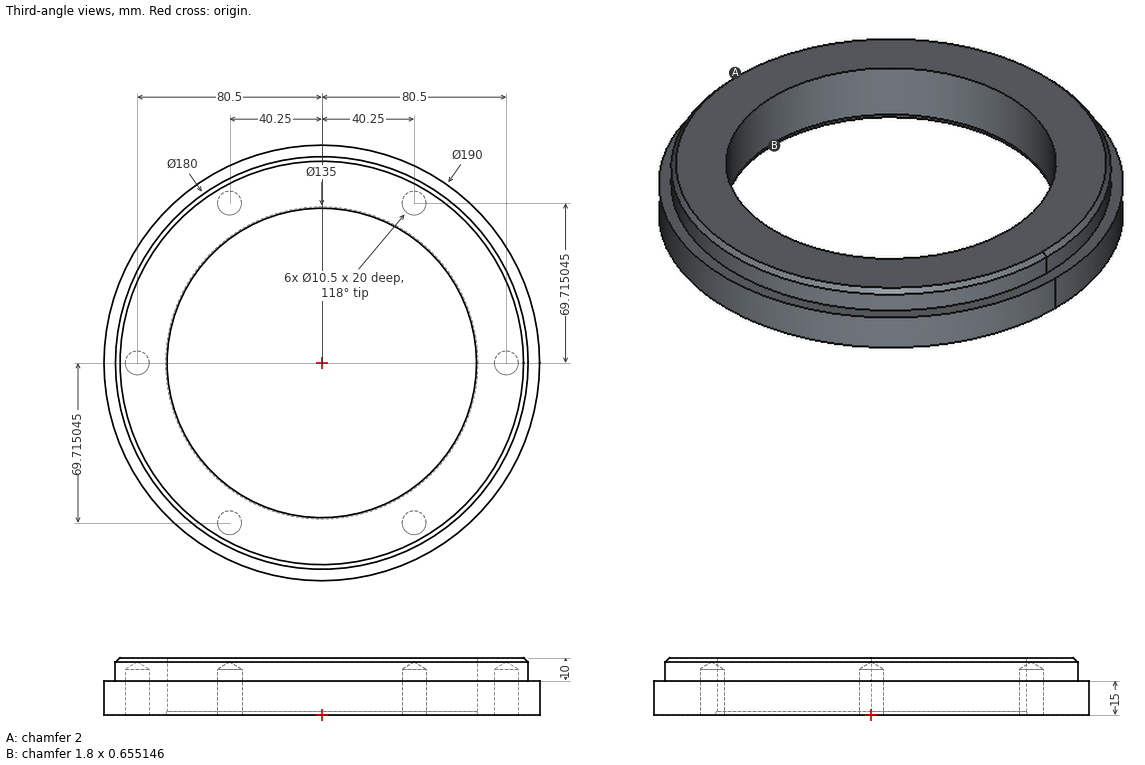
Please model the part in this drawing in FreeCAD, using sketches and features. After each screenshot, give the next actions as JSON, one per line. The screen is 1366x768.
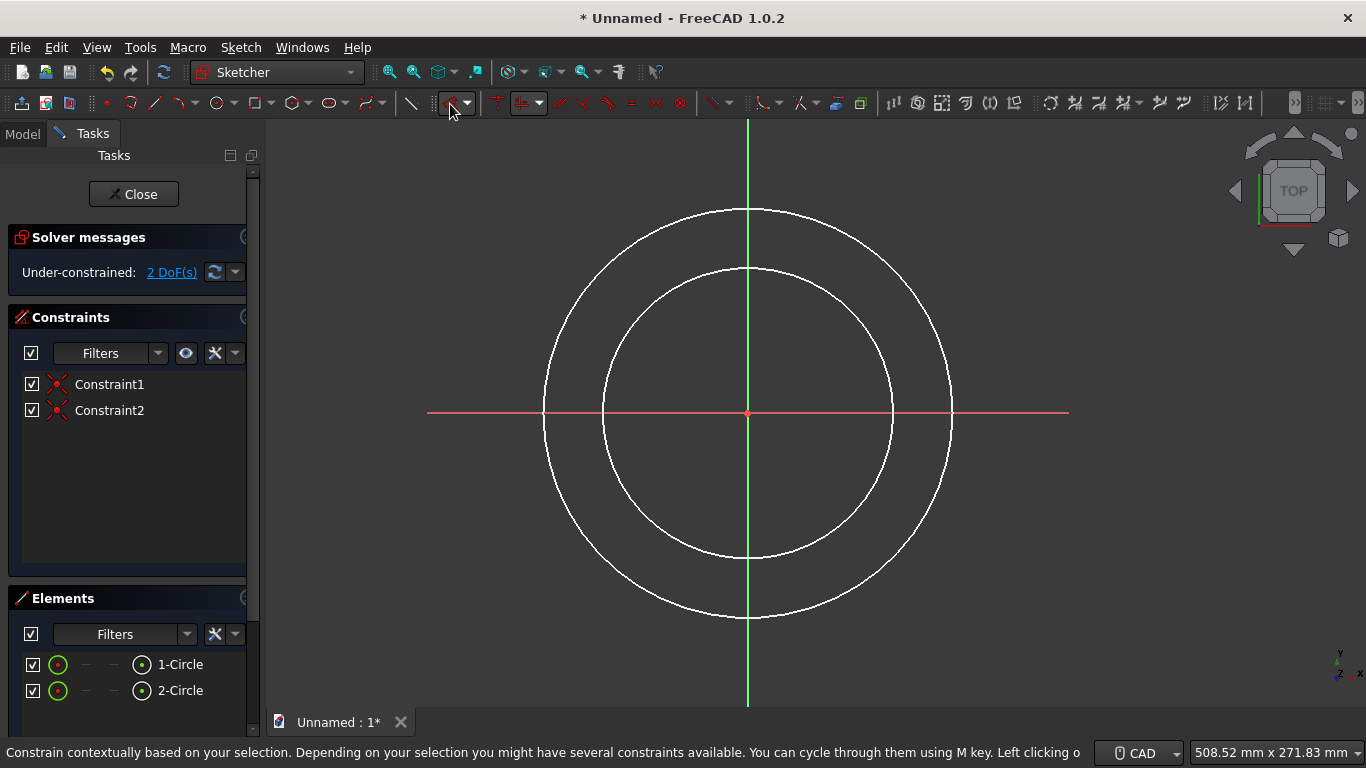
{"action": "left_click", "coordinate": [892, 268]}
{"action": "left_click", "coordinate": [915, 245]}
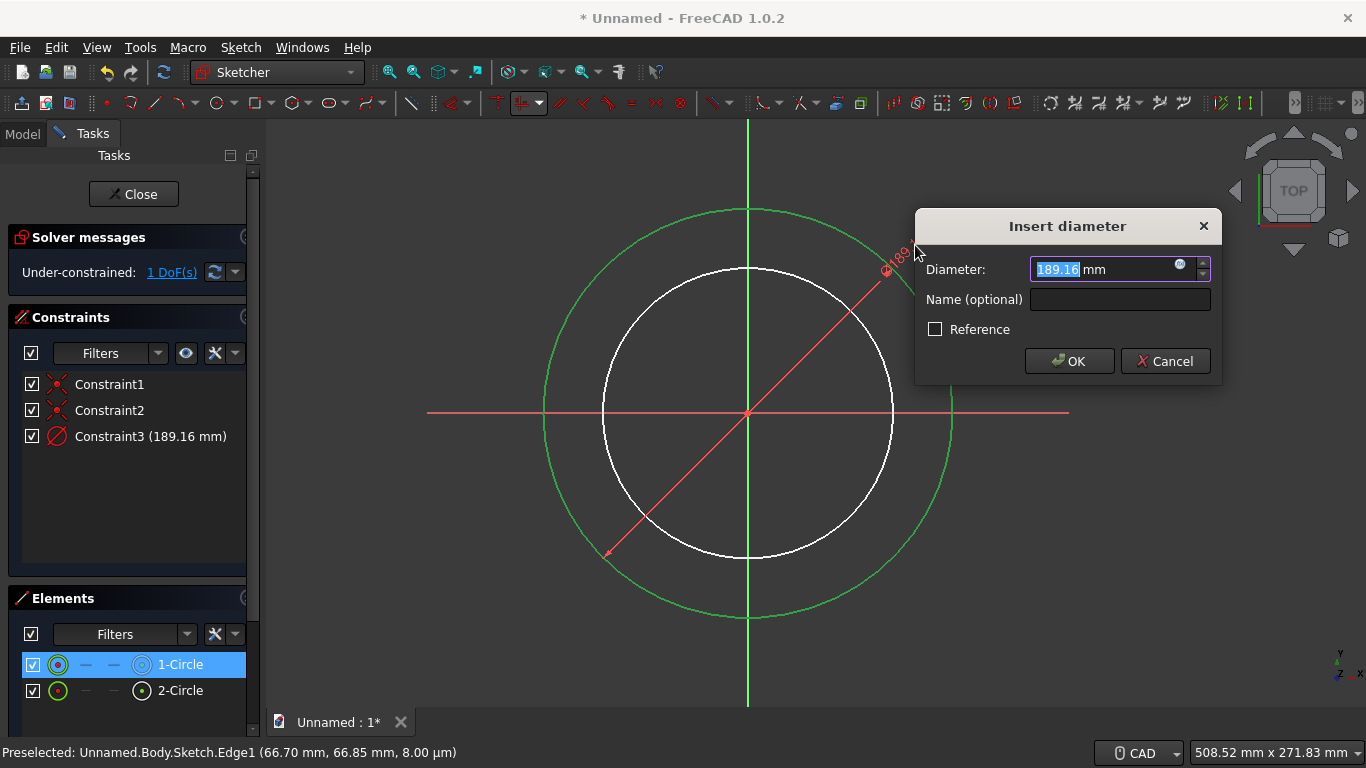
{"action": "type", "text": "190"}
{"action": "key", "text": "Return"}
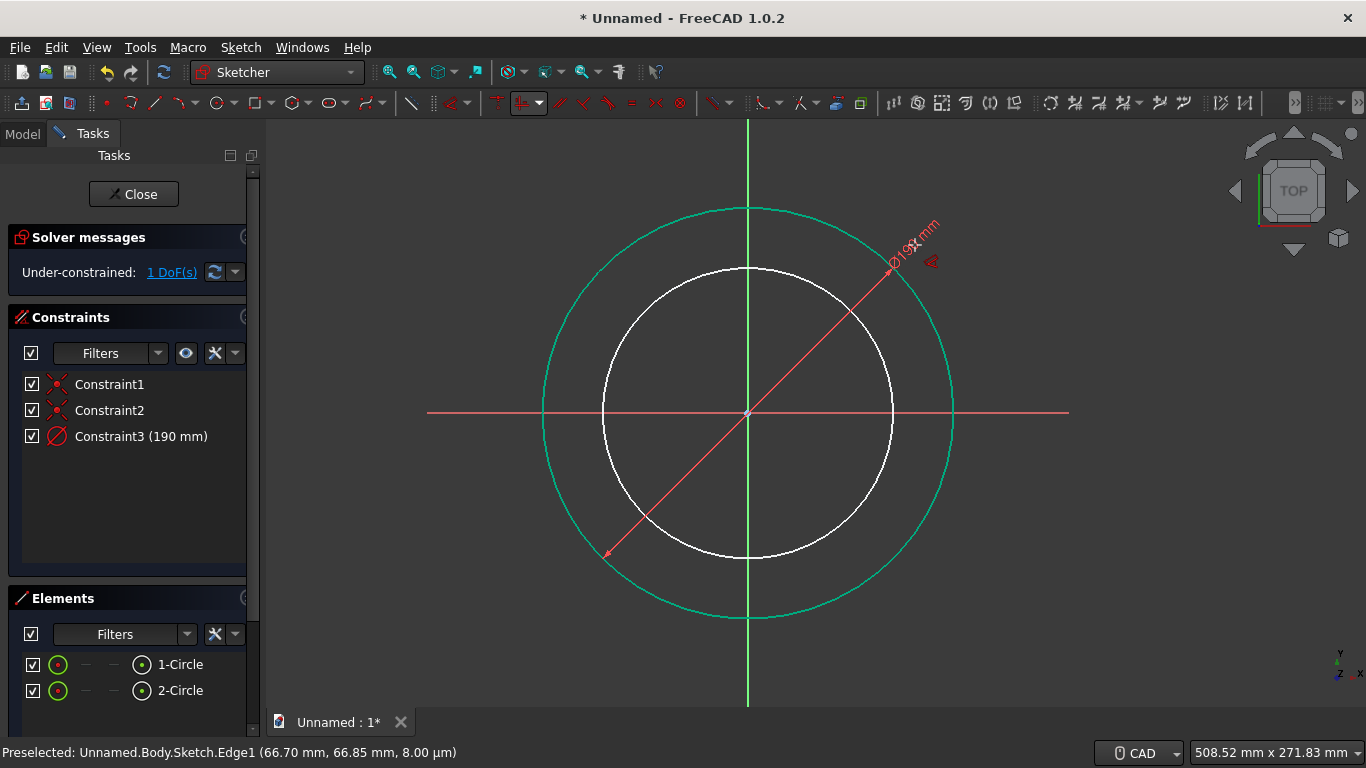
{"action": "left_click", "coordinate": [850, 310]}
{"action": "left_click", "coordinate": [872, 287]}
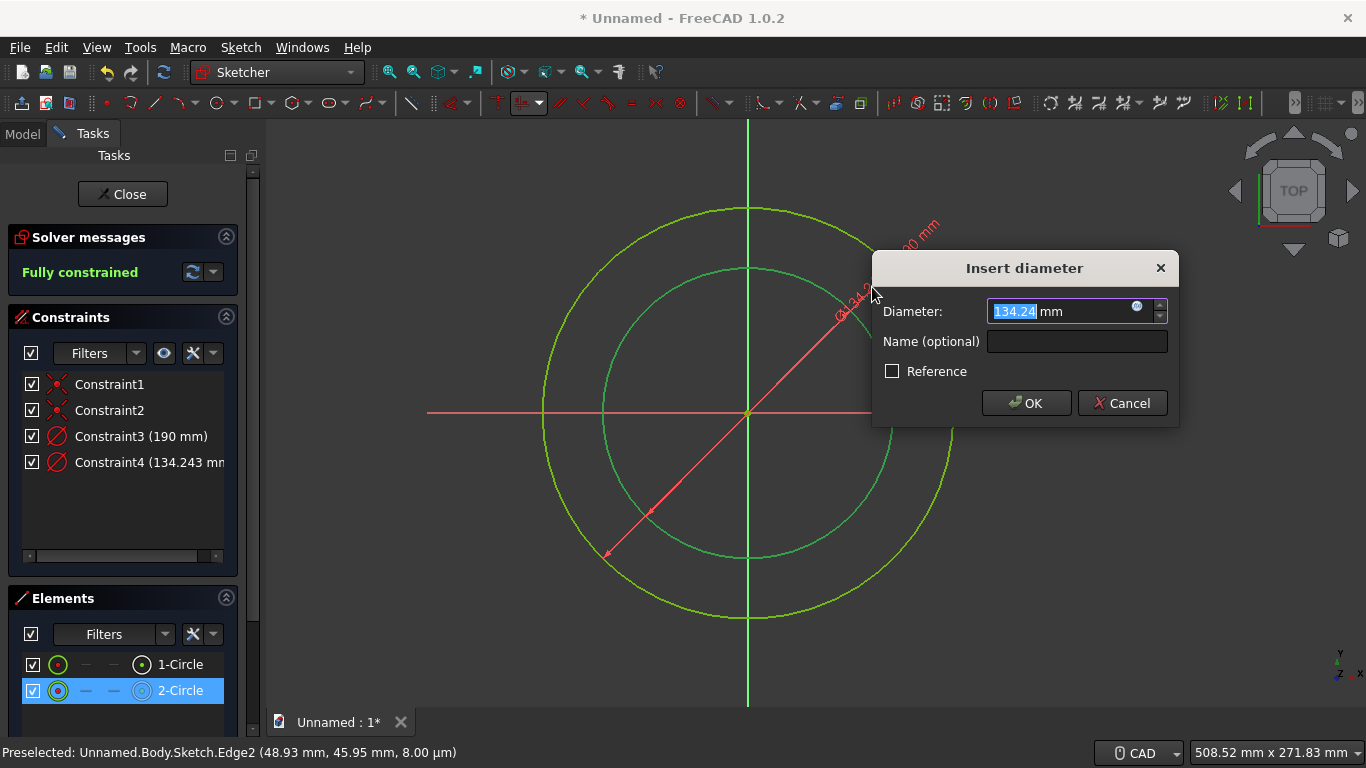
{"action": "type", "text": "135"}
{"action": "key", "text": "Return"}
{"action": "key", "text": "Escape"}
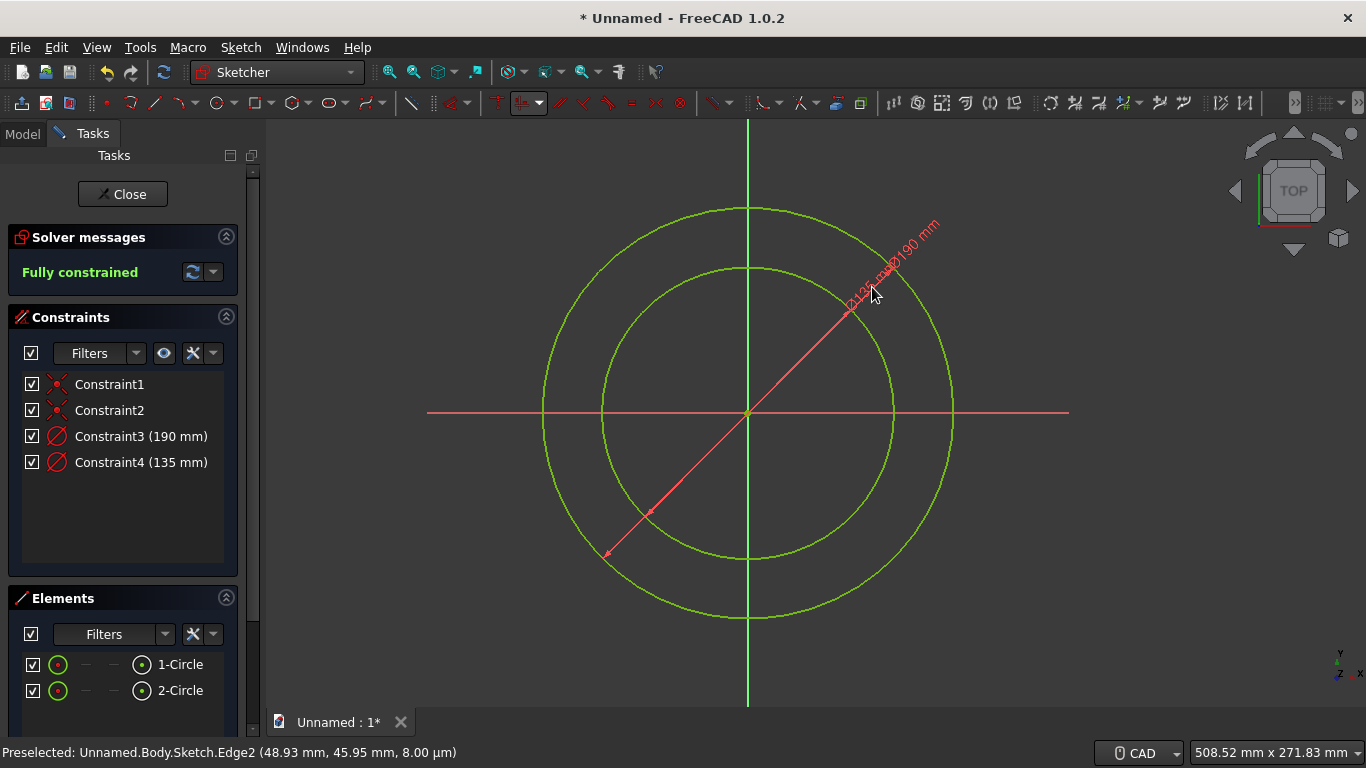
{"action": "left_click", "coordinate": [123, 194]}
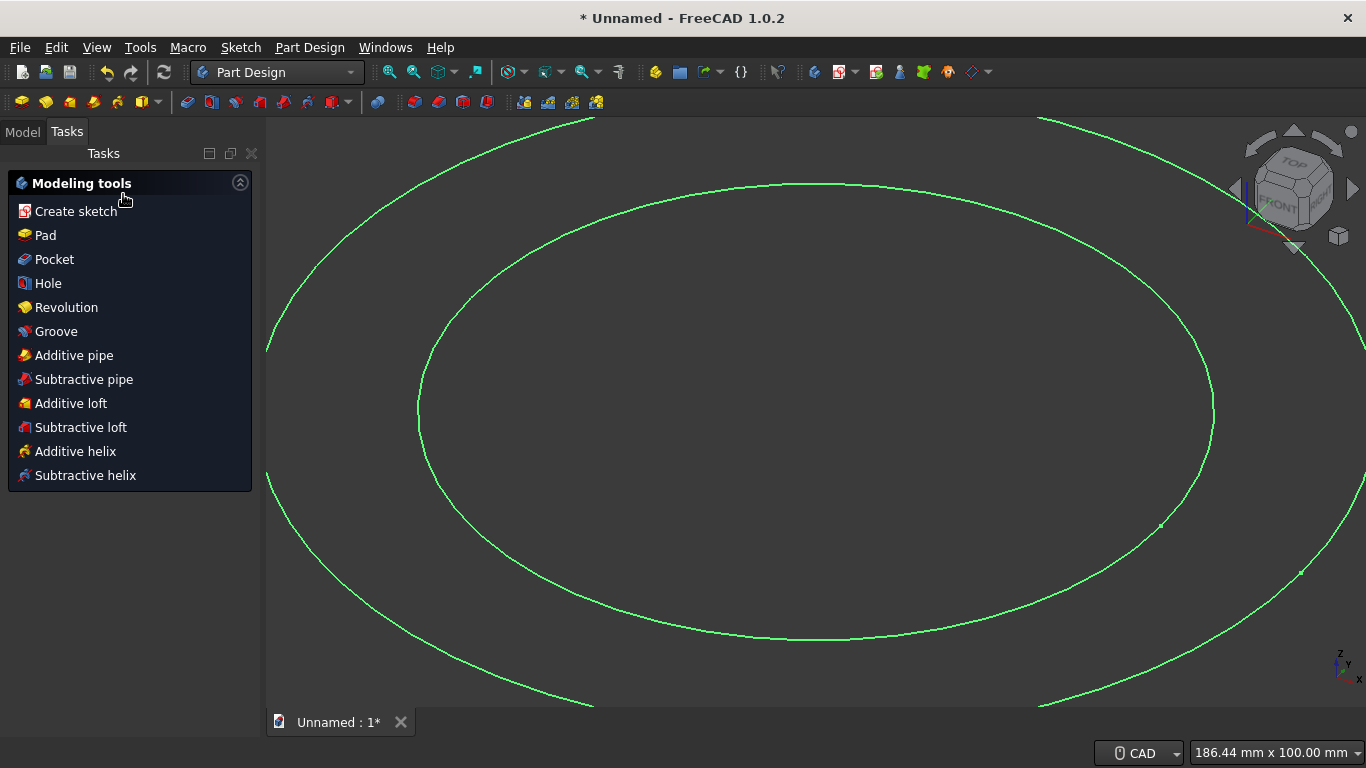
{"action": "left_click", "coordinate": [22, 102]}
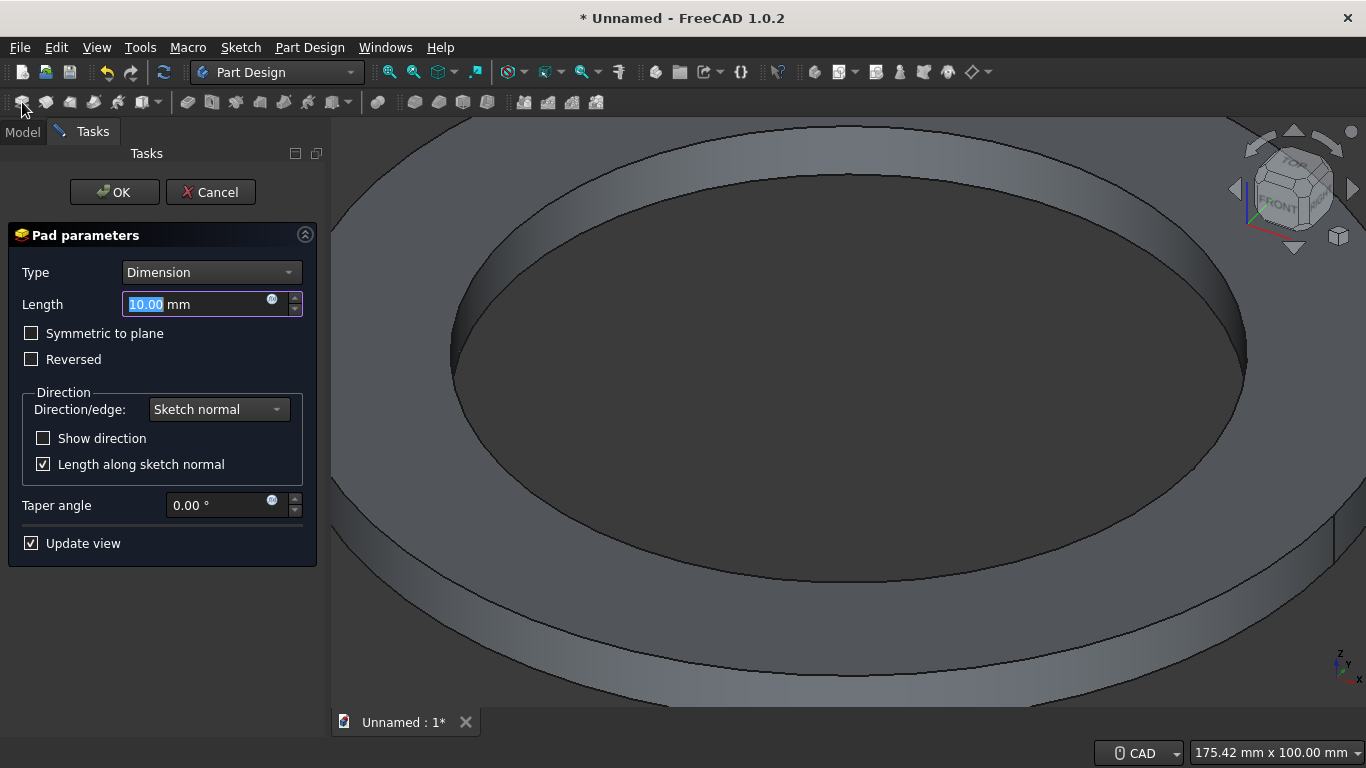
{"action": "type", "text": "15"}
{"action": "key", "text": "Tab"}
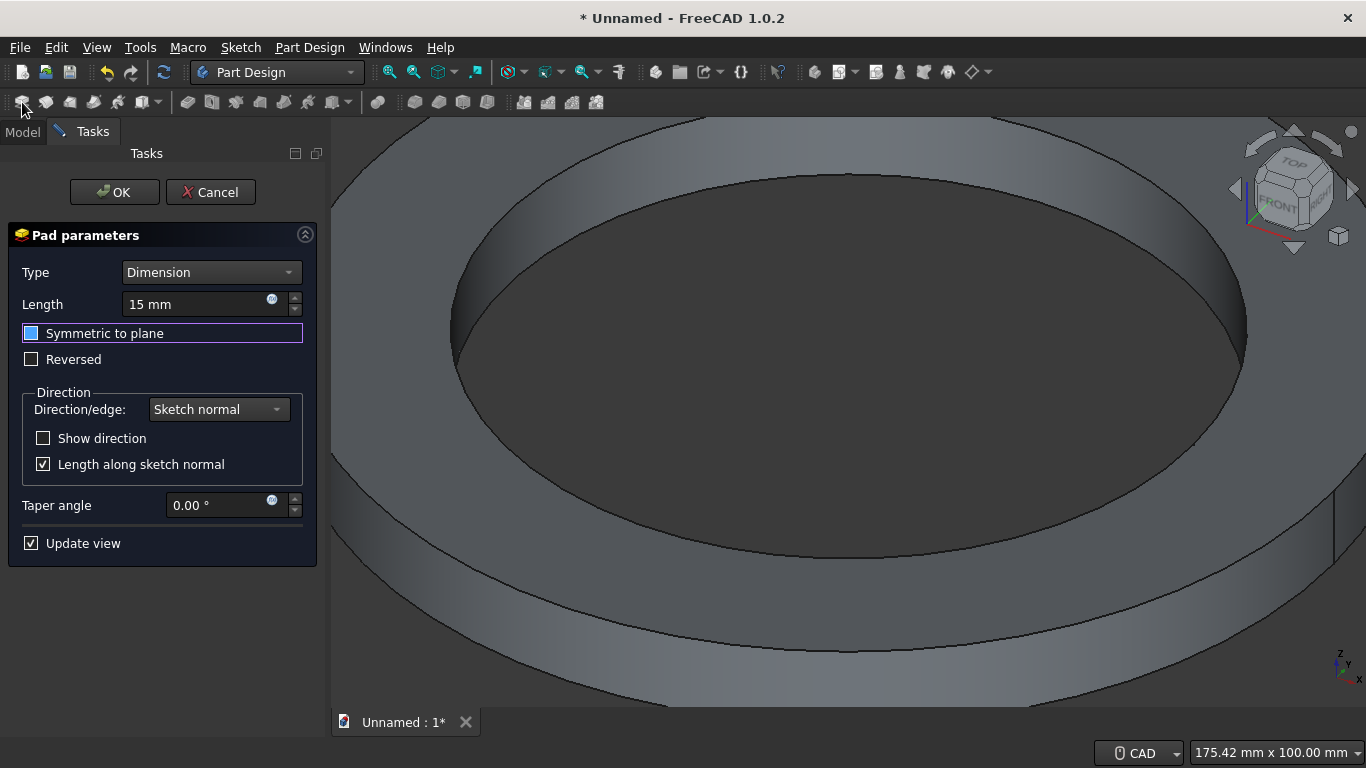
{"action": "left_click", "coordinate": [115, 192]}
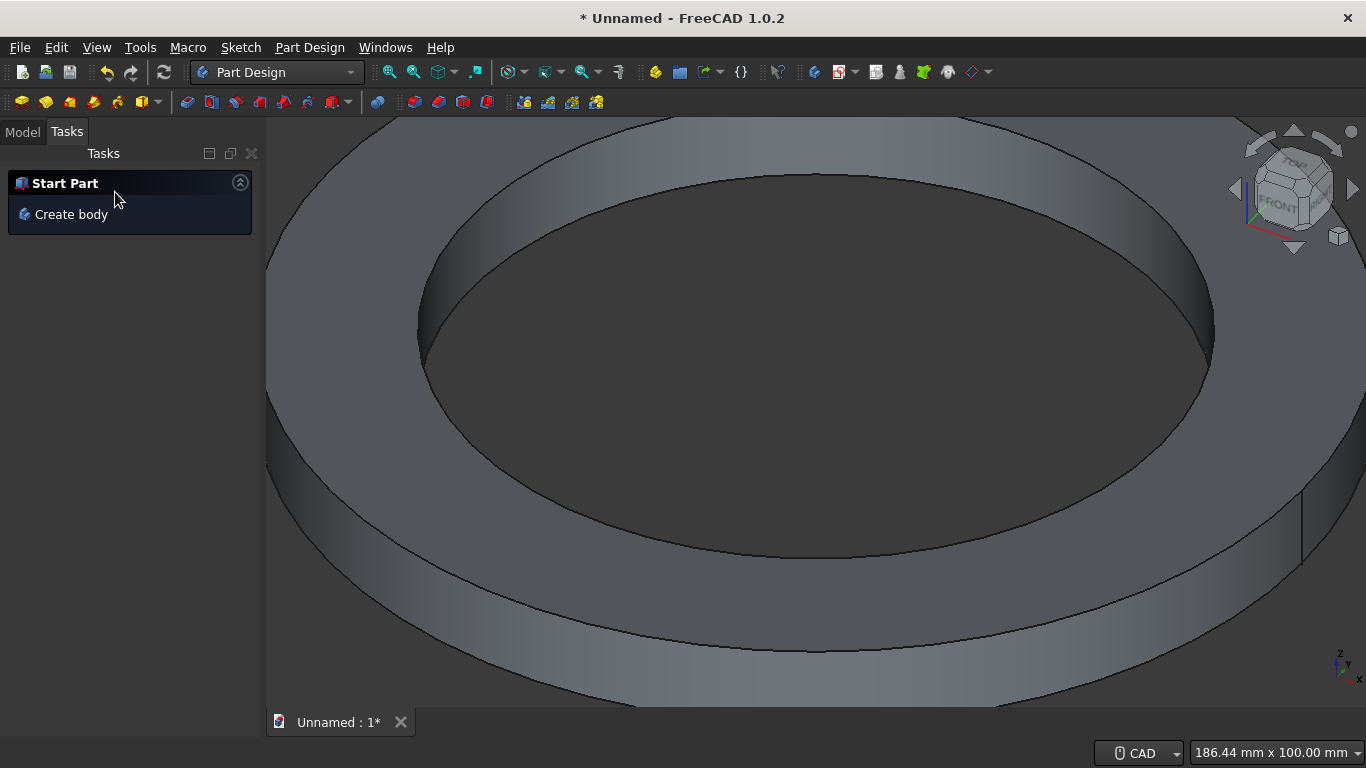
{"action": "left_click", "coordinate": [390, 72]}